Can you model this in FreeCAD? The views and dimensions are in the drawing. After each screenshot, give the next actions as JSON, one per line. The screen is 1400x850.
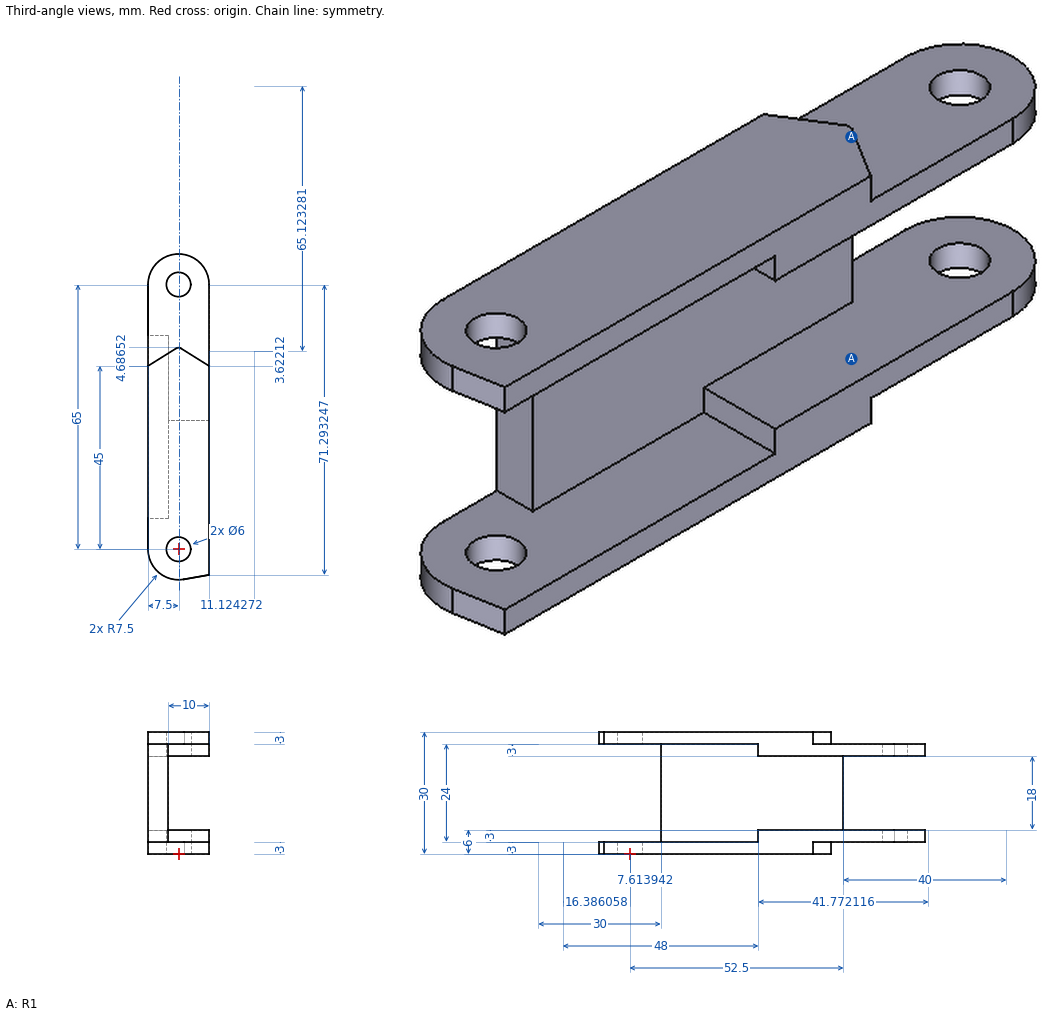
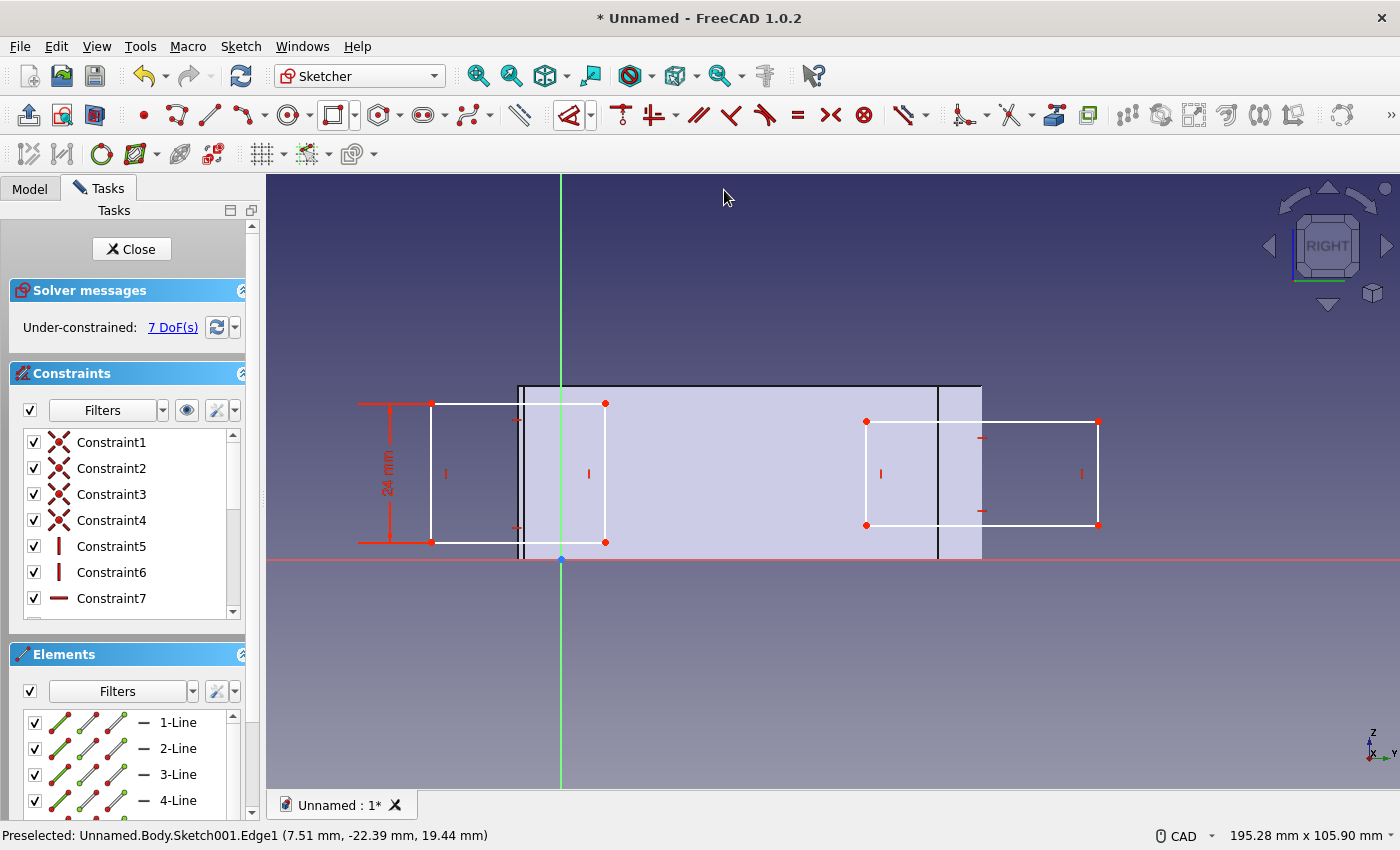
{"action": "left_click", "coordinate": [483, 543]}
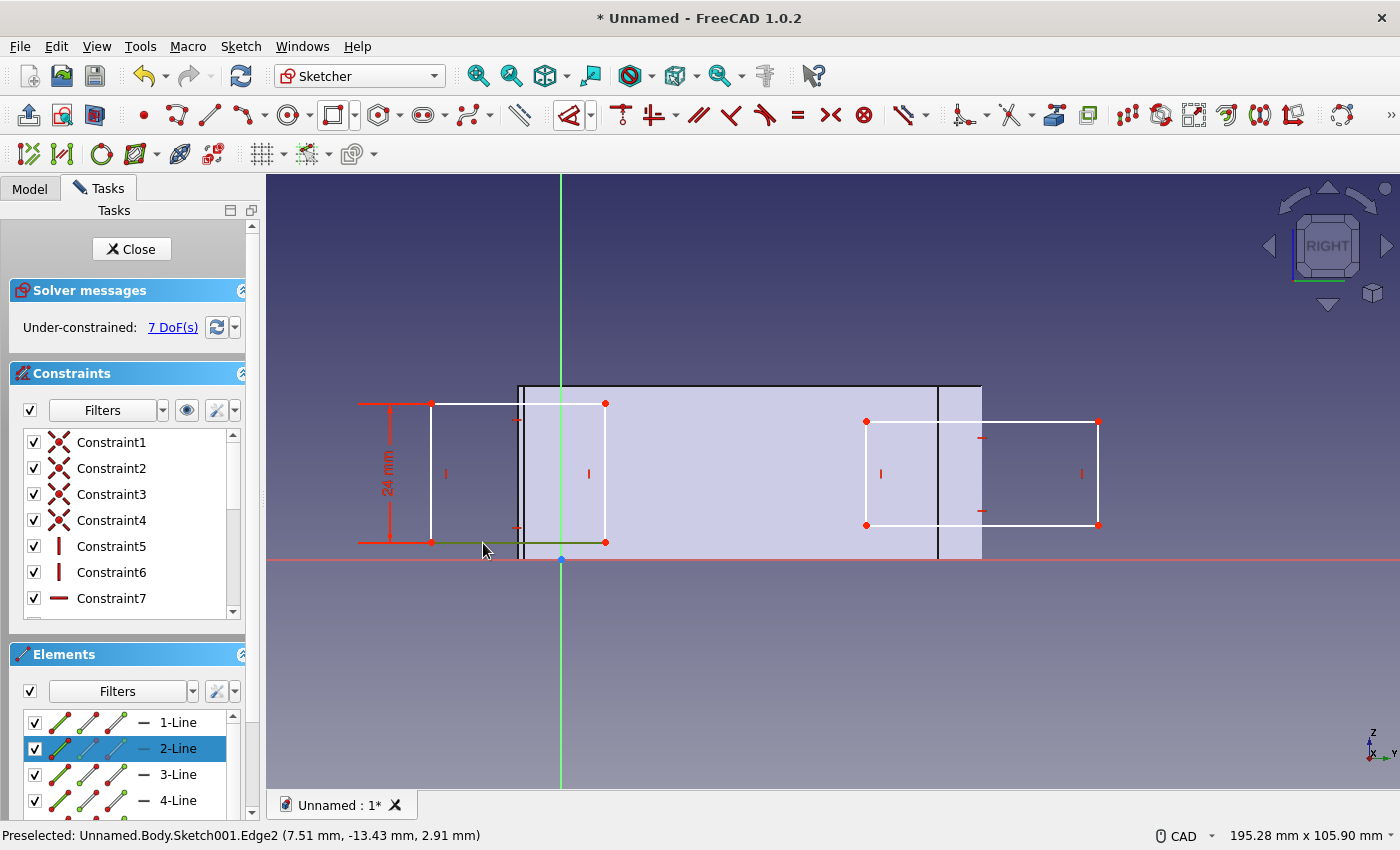
{"action": "key", "text": "l"}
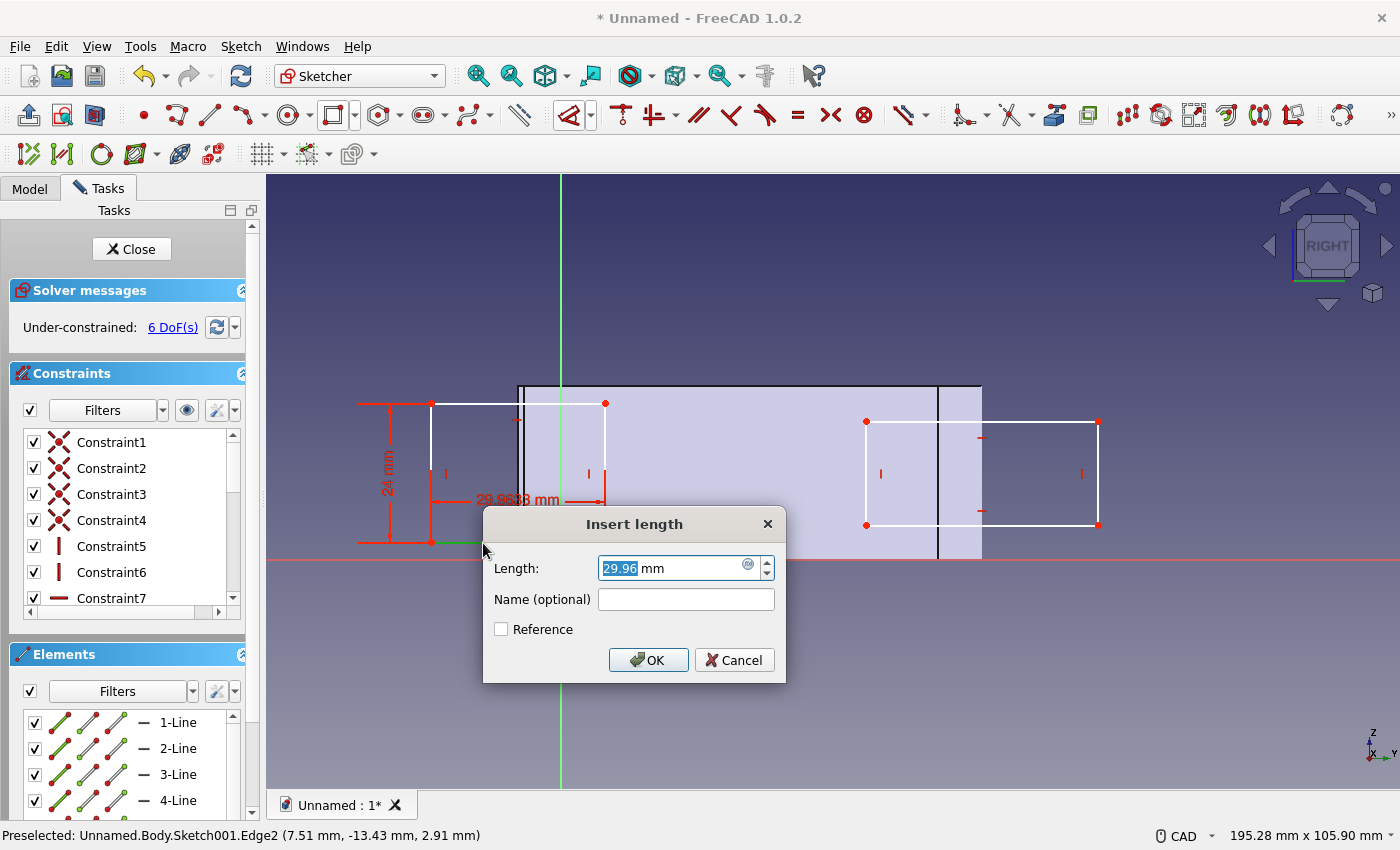
{"action": "type", "text": "30"}
{"action": "key", "text": "Return"}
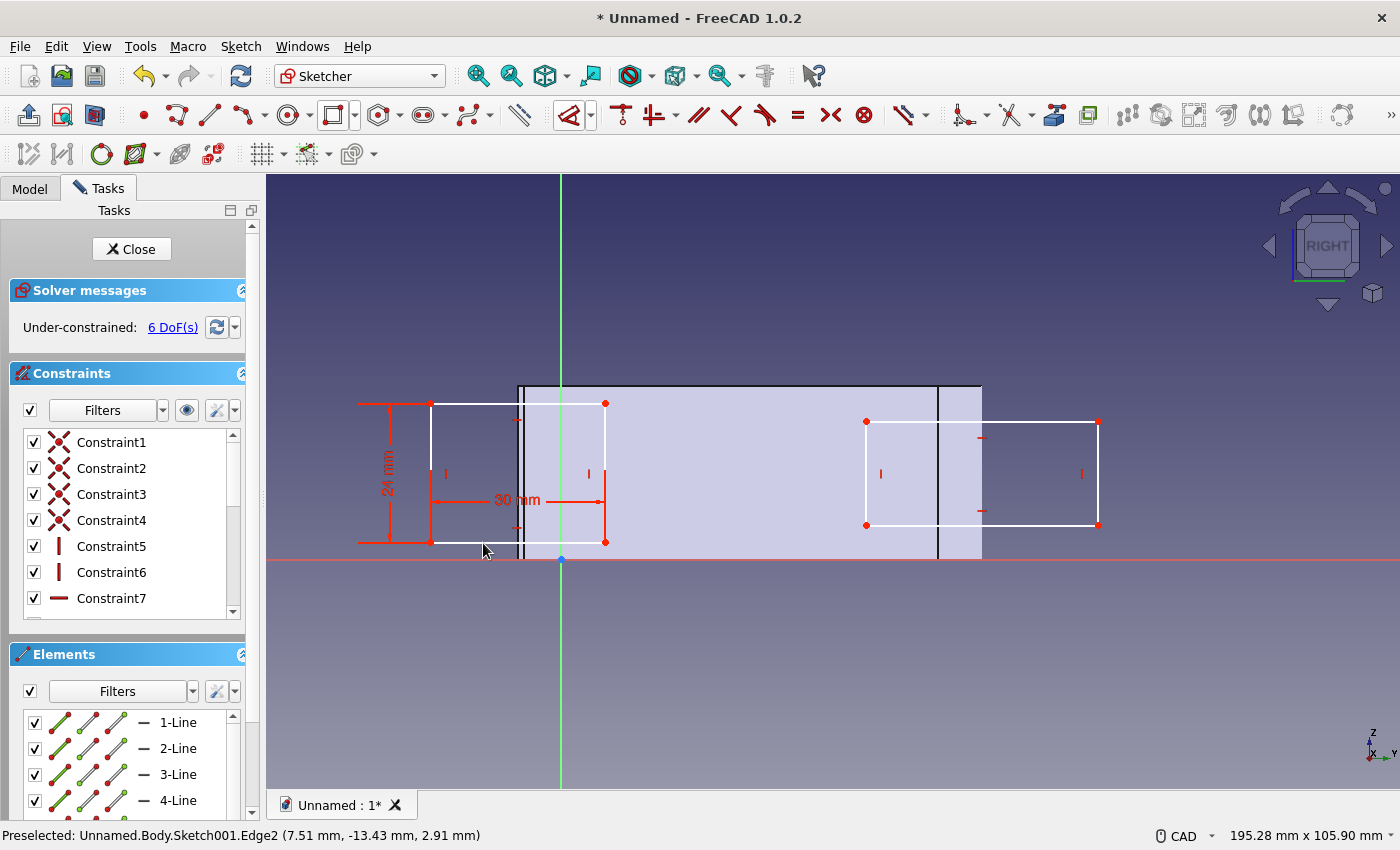
{"action": "left_click", "coordinate": [866, 453]}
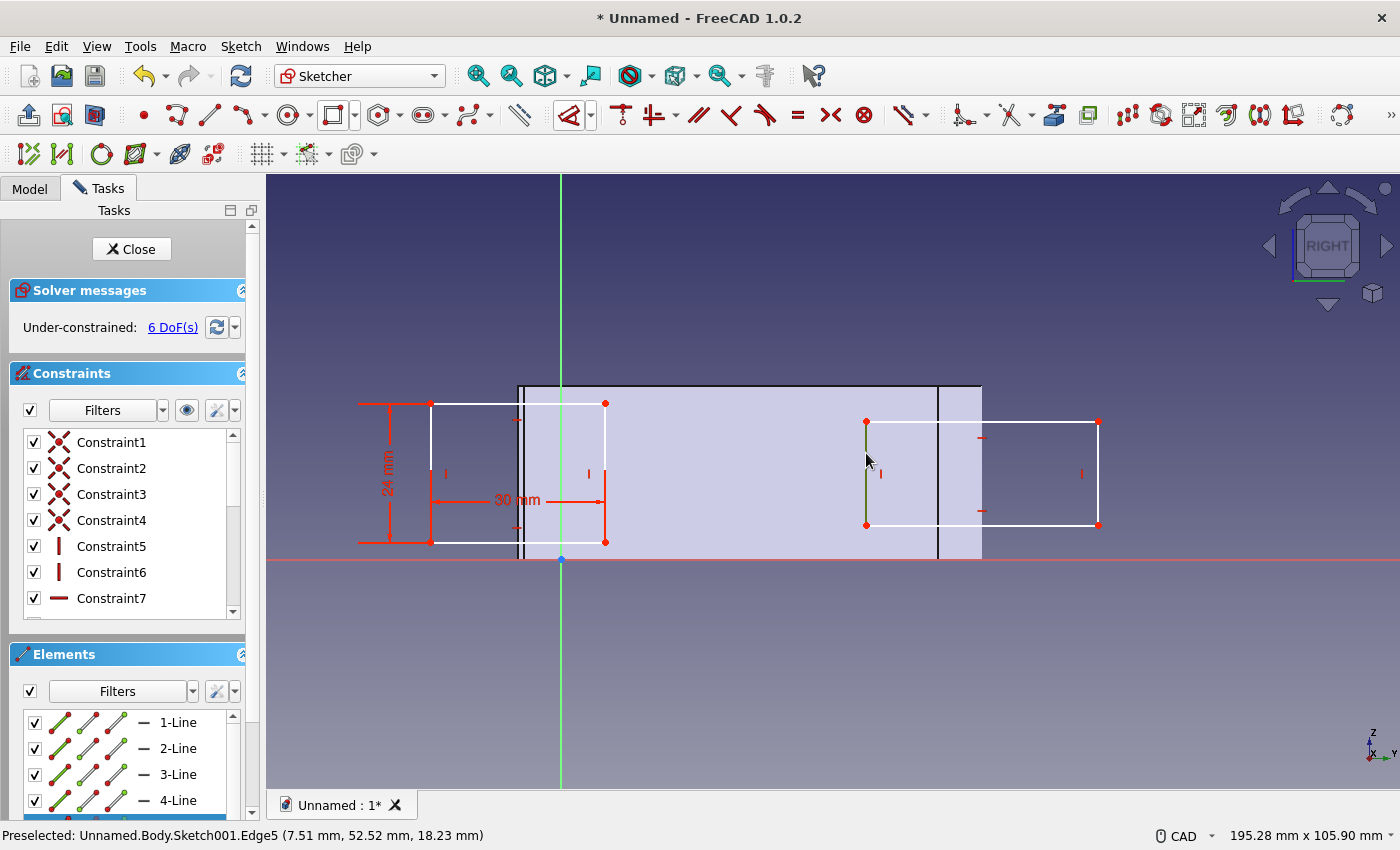
{"action": "key", "text": "i"}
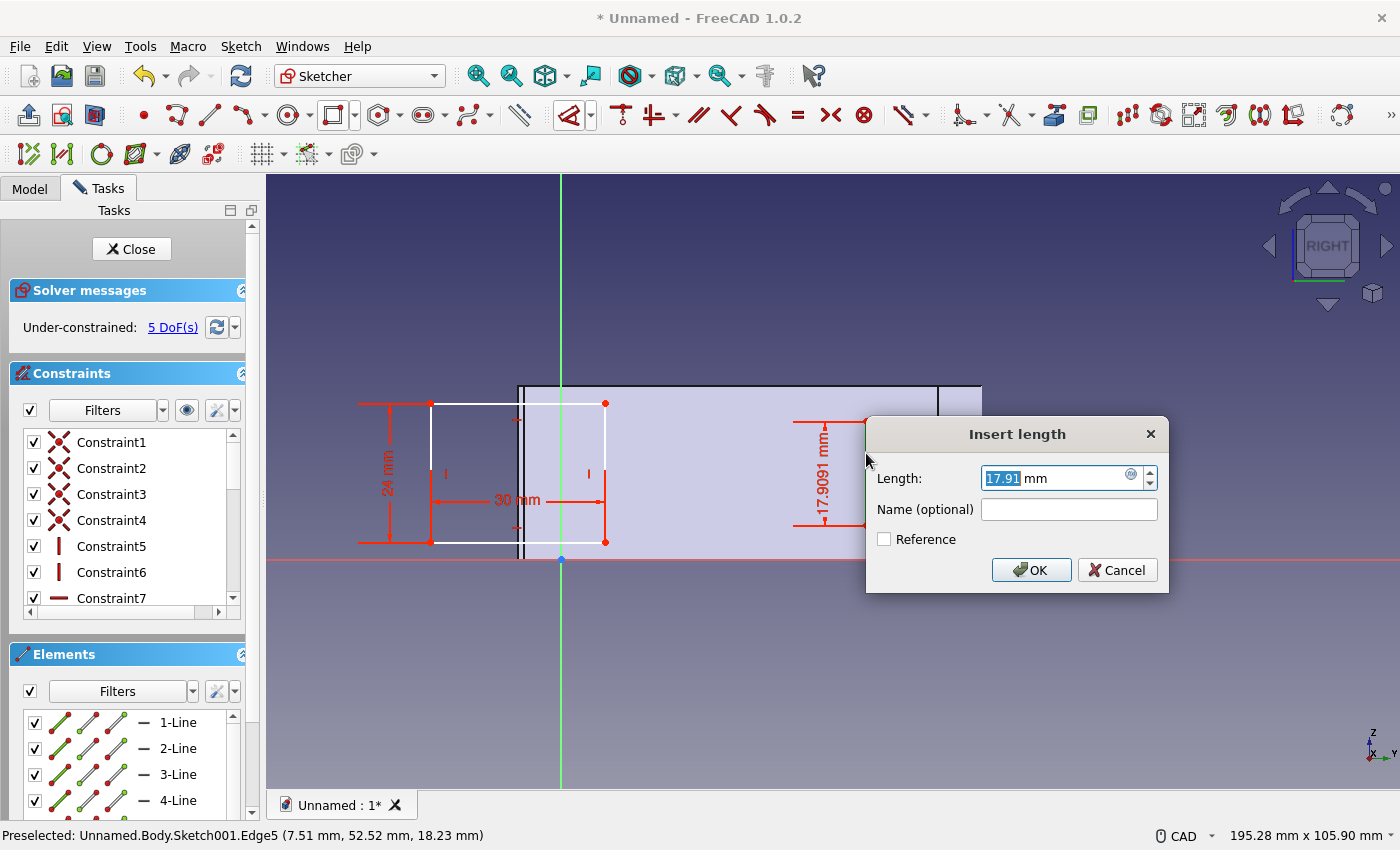
{"action": "type", "text": "18"}
{"action": "key", "text": "Return"}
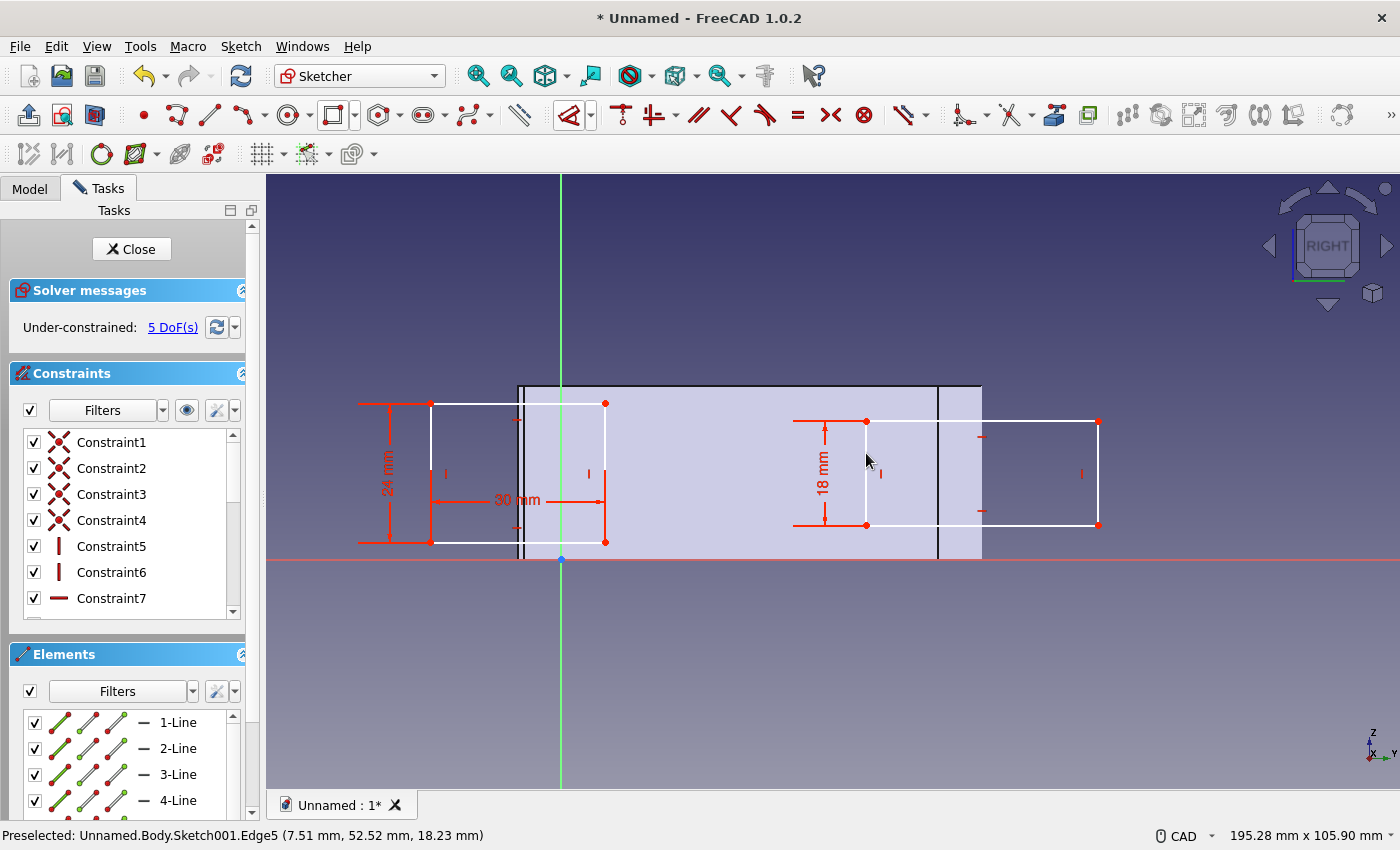
{"action": "left_click", "coordinate": [936, 526]}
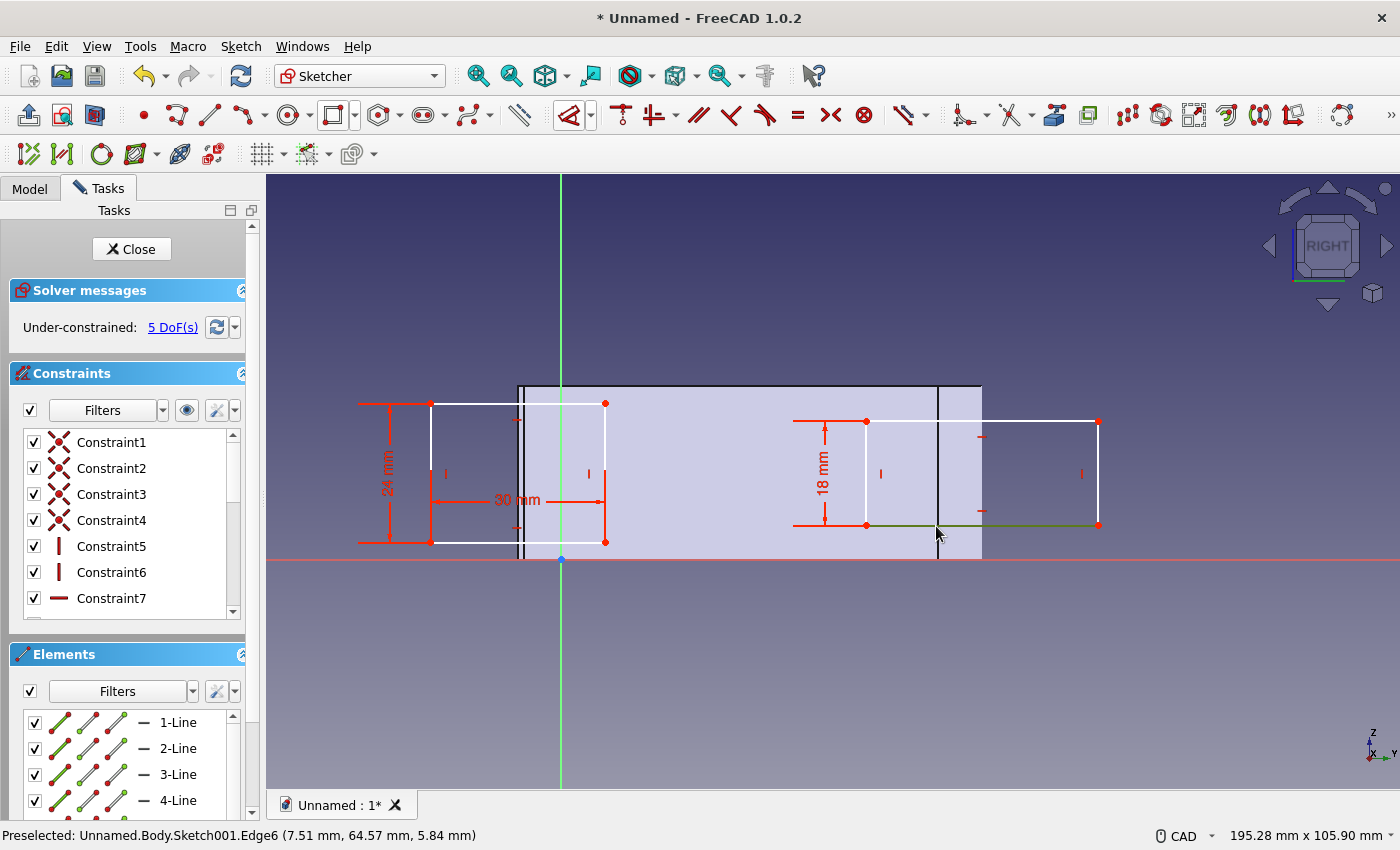
{"action": "key", "text": "l"}